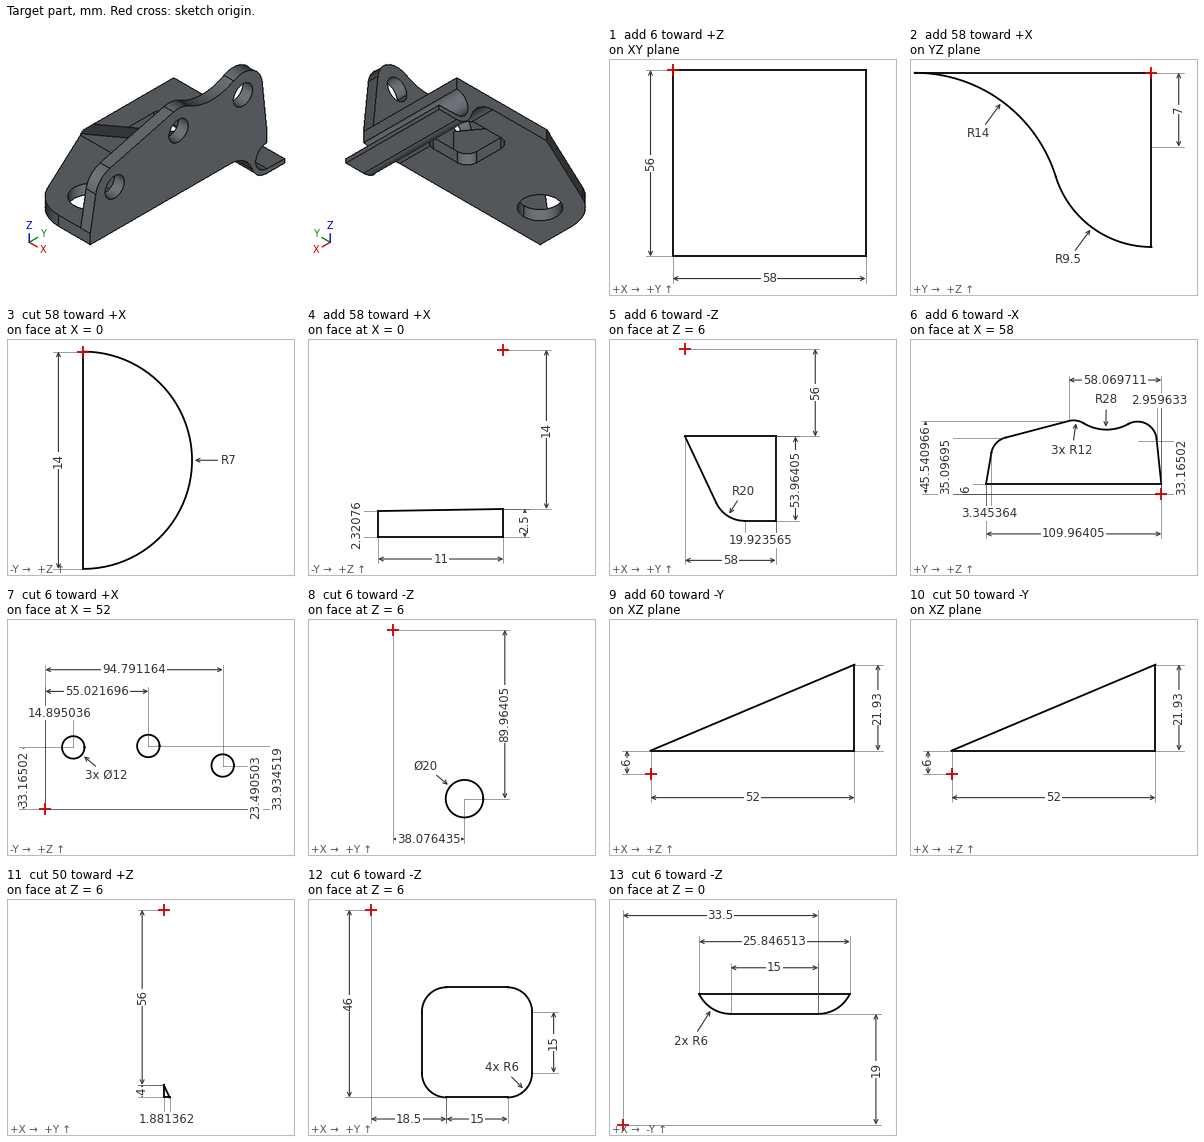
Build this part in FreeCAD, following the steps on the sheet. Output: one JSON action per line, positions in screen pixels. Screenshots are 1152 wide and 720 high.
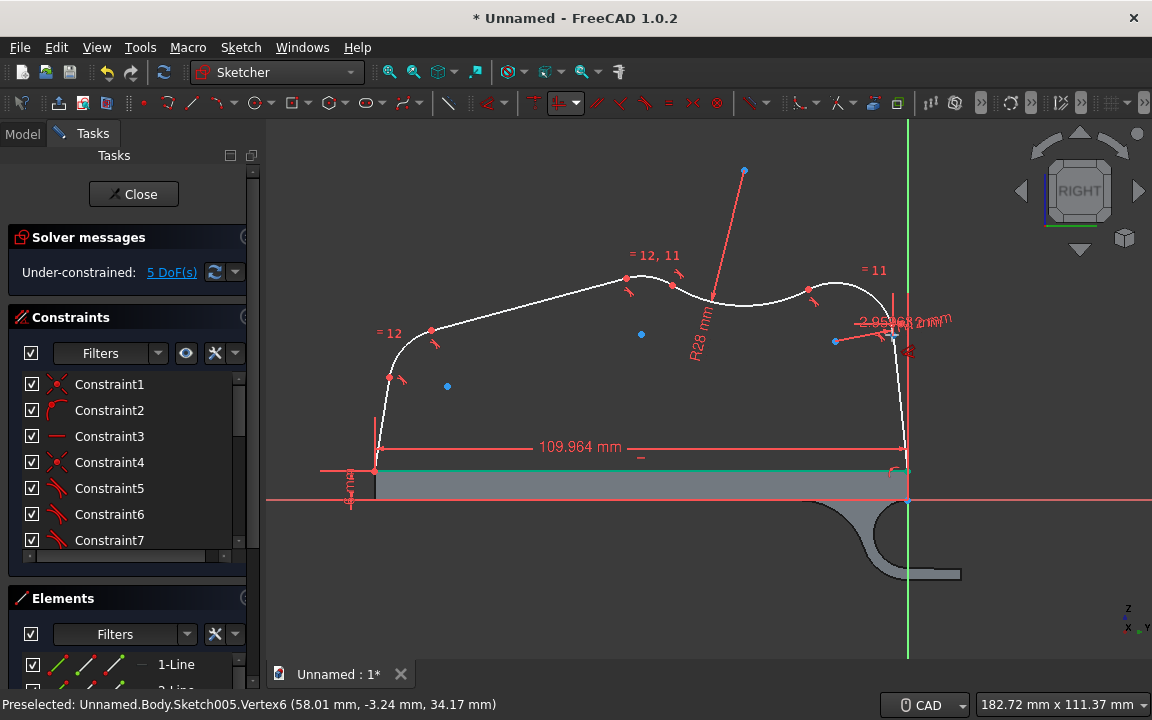
{"action": "left_click", "coordinate": [432, 331]}
{"action": "left_click", "coordinate": [942, 415]}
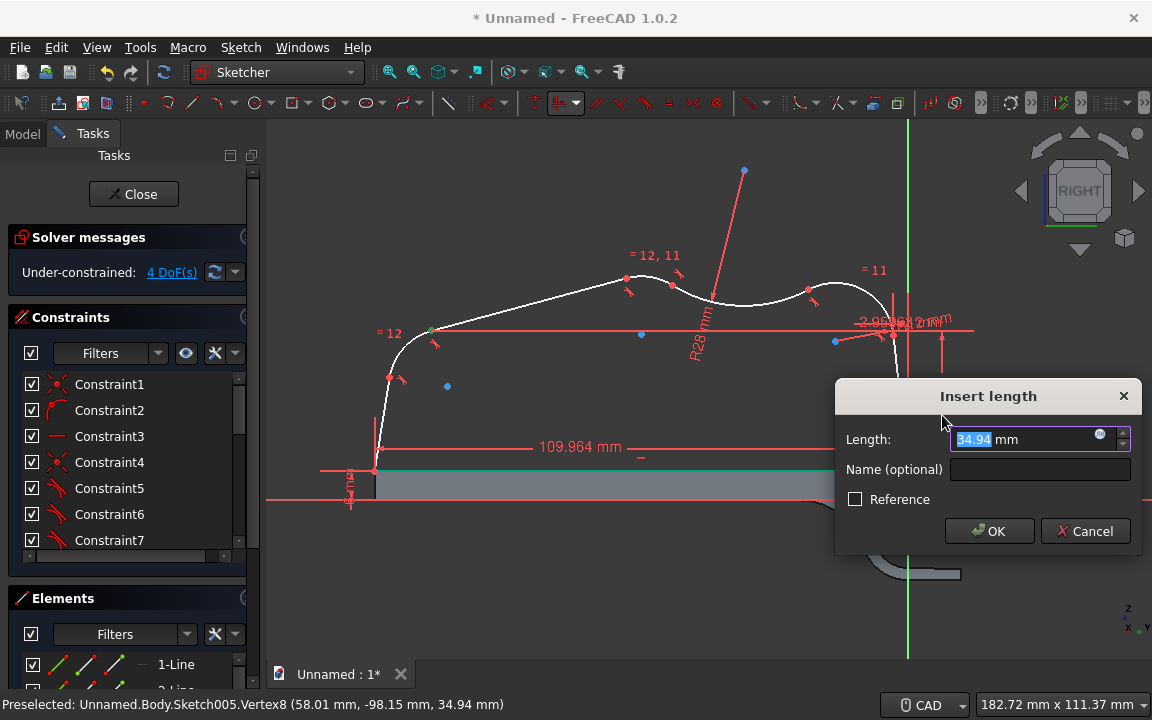
{"action": "type", "text": "35.09695"}
{"action": "key", "text": "Return"}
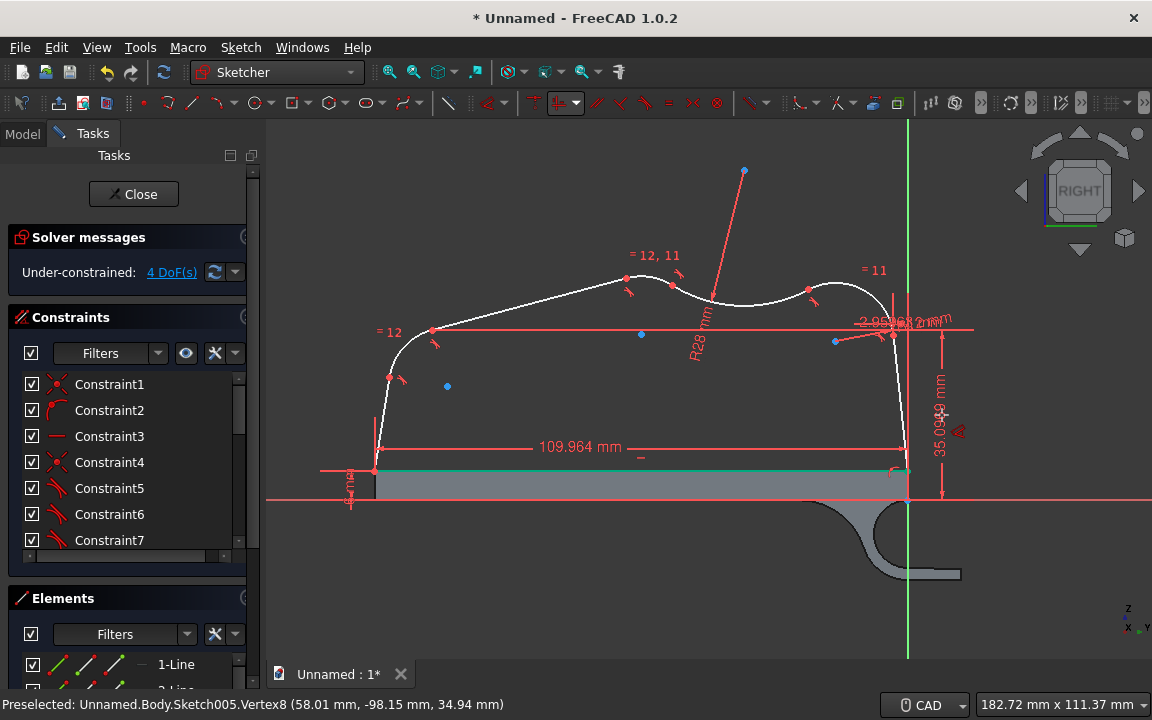
{"action": "scroll", "coordinate": [385, 405], "scroll_direction": "up", "scroll_amount": 5}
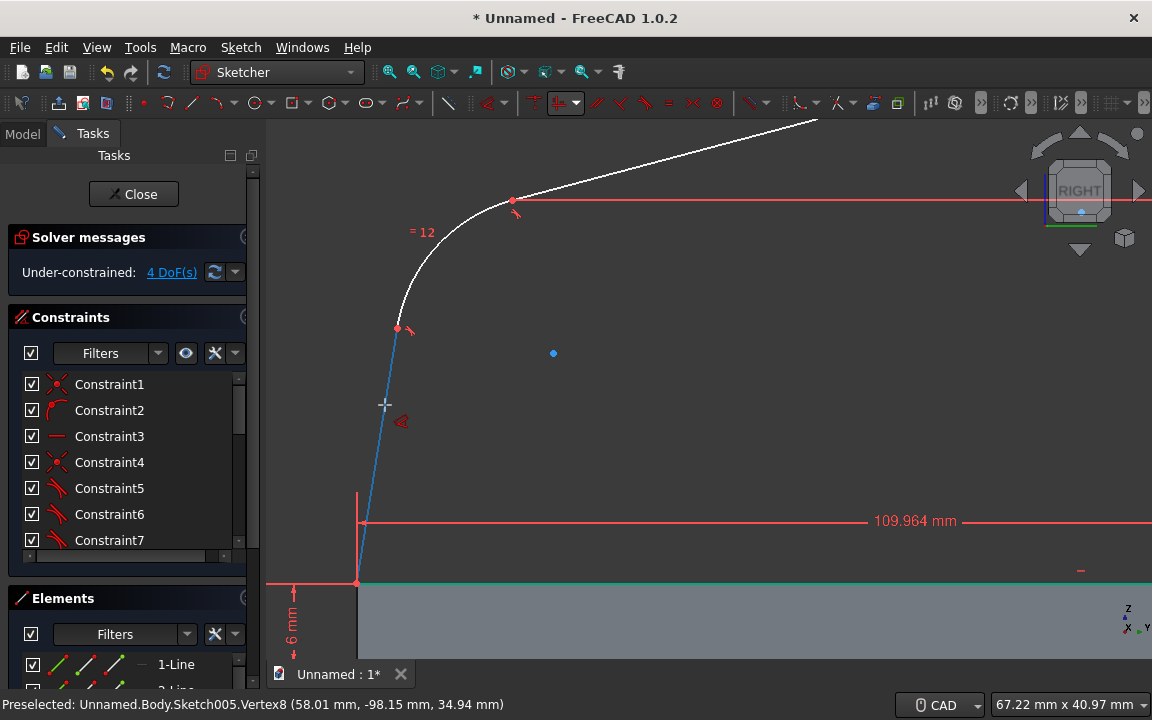
{"action": "left_click", "coordinate": [385, 405]}
{"action": "left_click", "coordinate": [377, 618]}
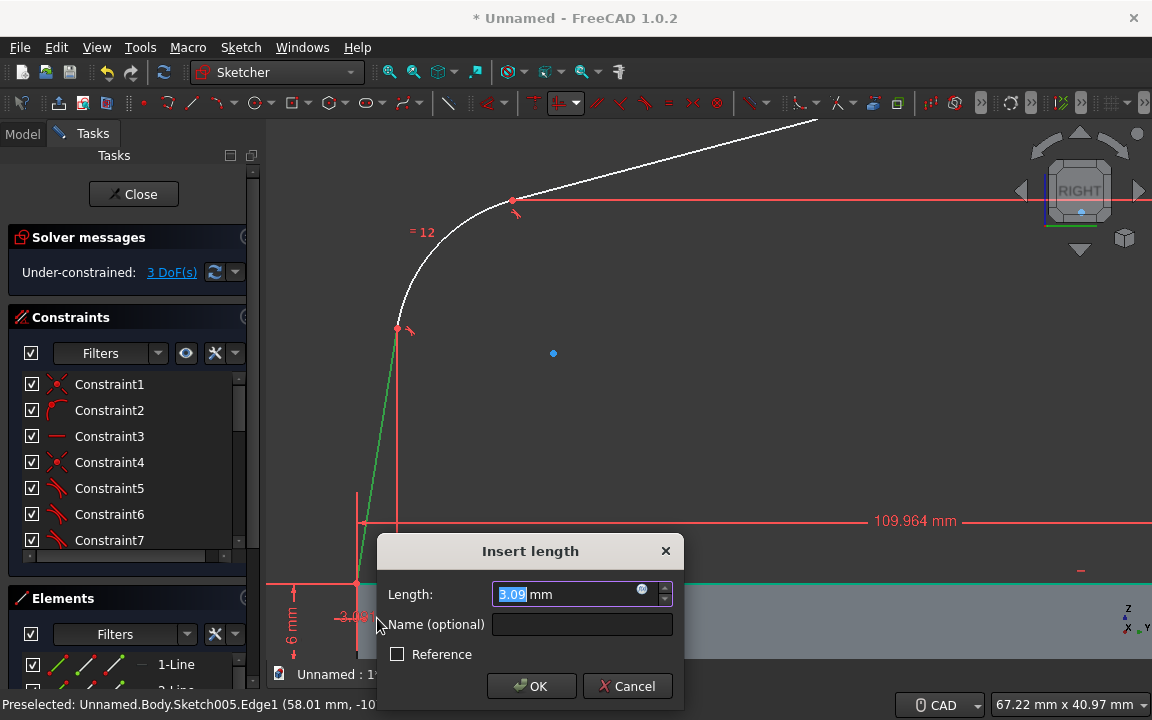
{"action": "type", "text": "3.345364"}
{"action": "key", "text": "Return"}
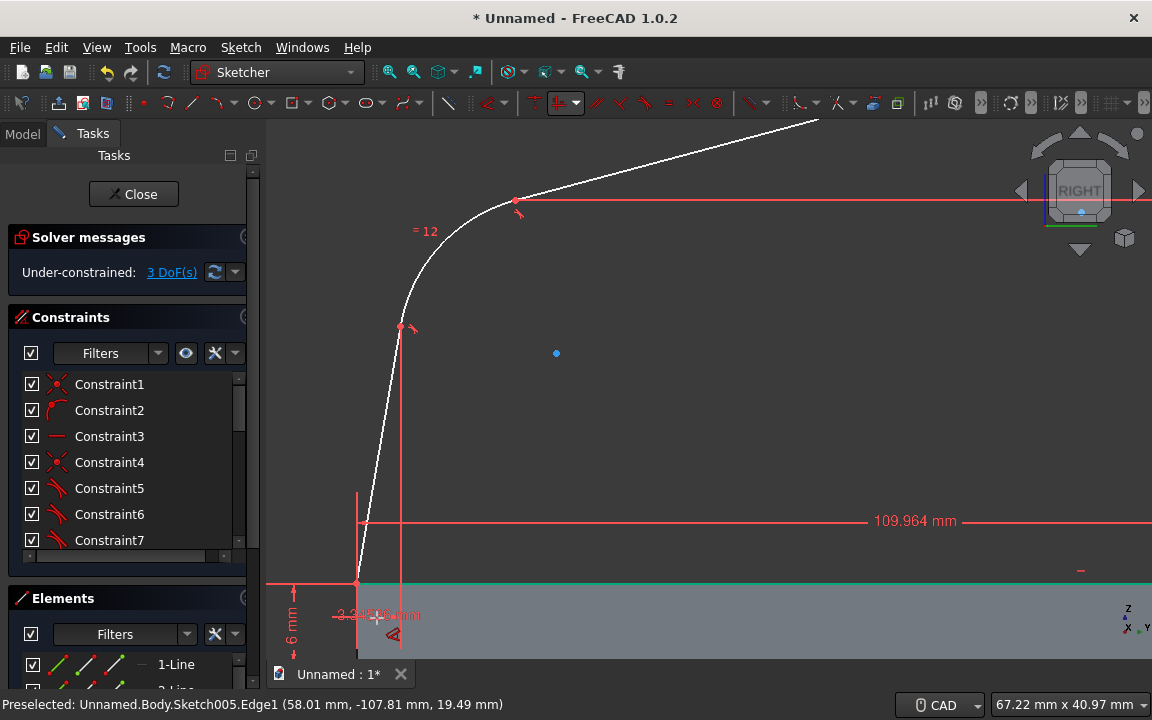
{"action": "scroll", "coordinate": [384, 405], "scroll_direction": "down", "scroll_amount": 5}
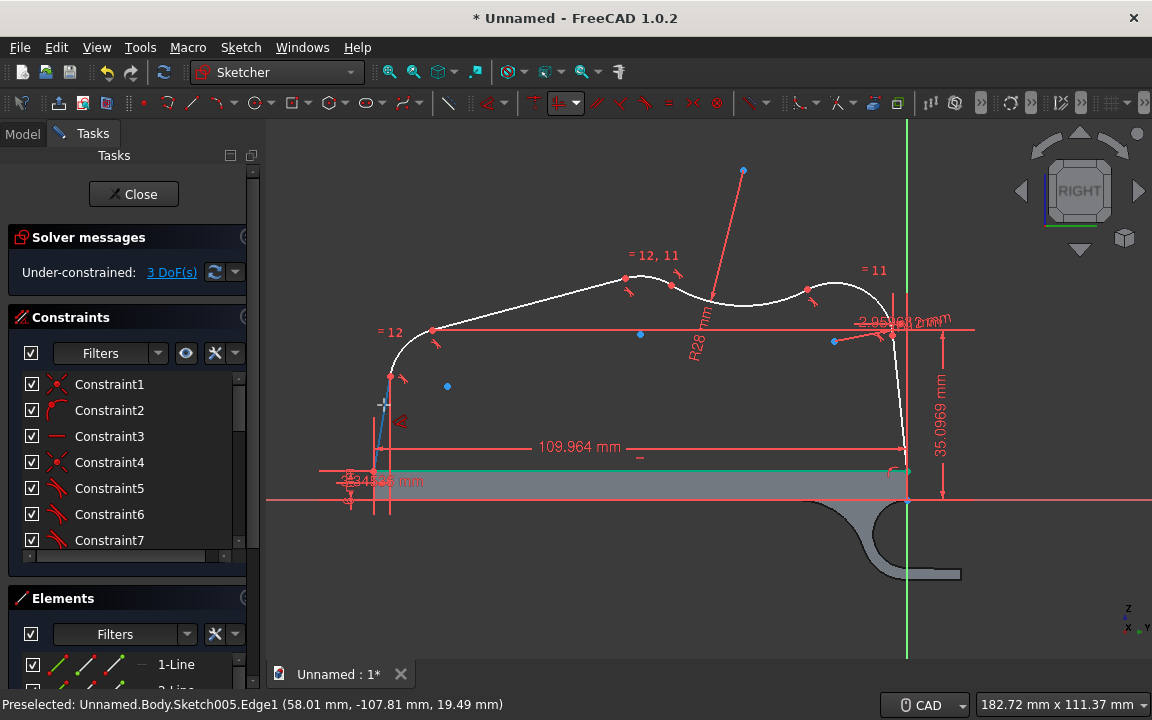
{"action": "left_click", "coordinate": [835, 341]}
{"action": "left_click", "coordinate": [941, 384]}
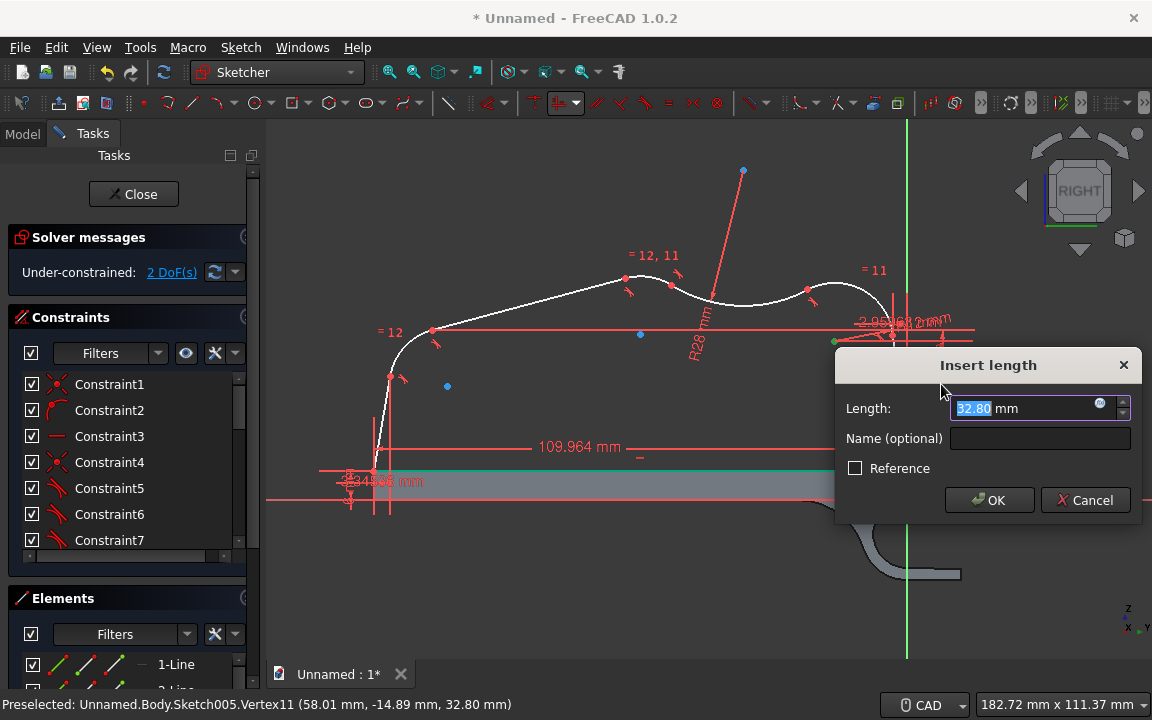
{"action": "type", "text": "33.16502"}
{"action": "key", "text": "Return"}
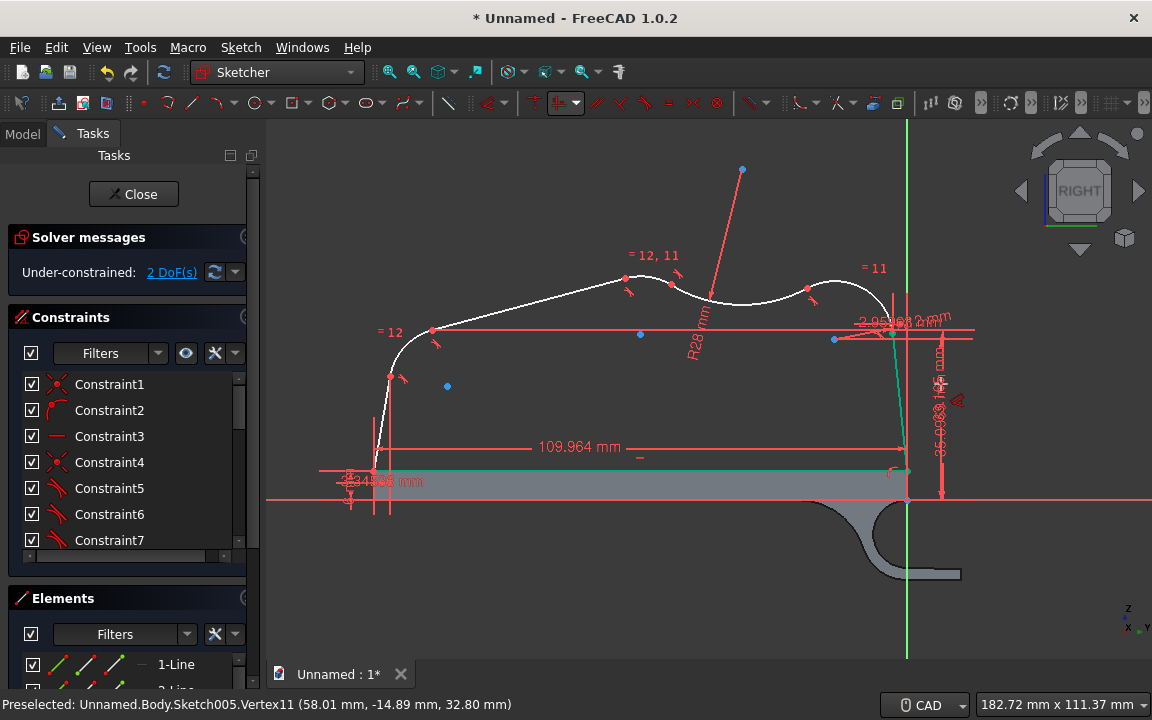
{"action": "left_click", "coordinate": [626, 278]}
{"action": "left_click", "coordinate": [766, 534]}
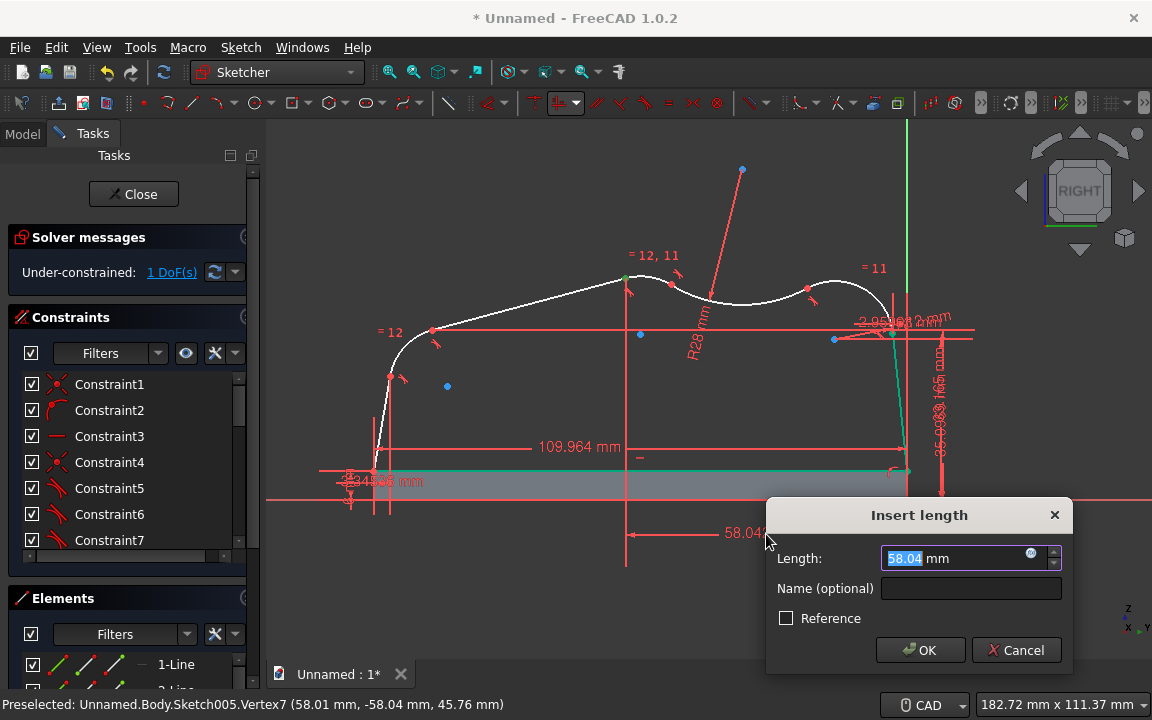
{"action": "type", "text": "58.069711"}
{"action": "key", "text": "Return"}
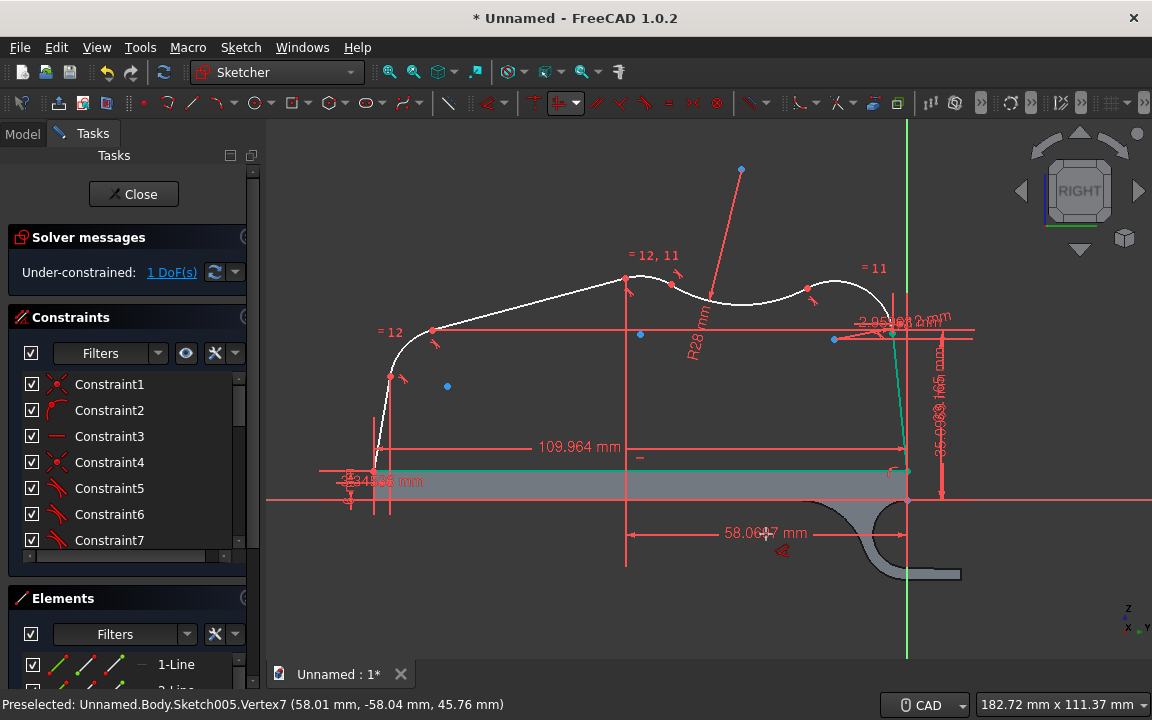
{"action": "left_click", "coordinate": [626, 278]}
{"action": "left_click", "coordinate": [941, 440]}